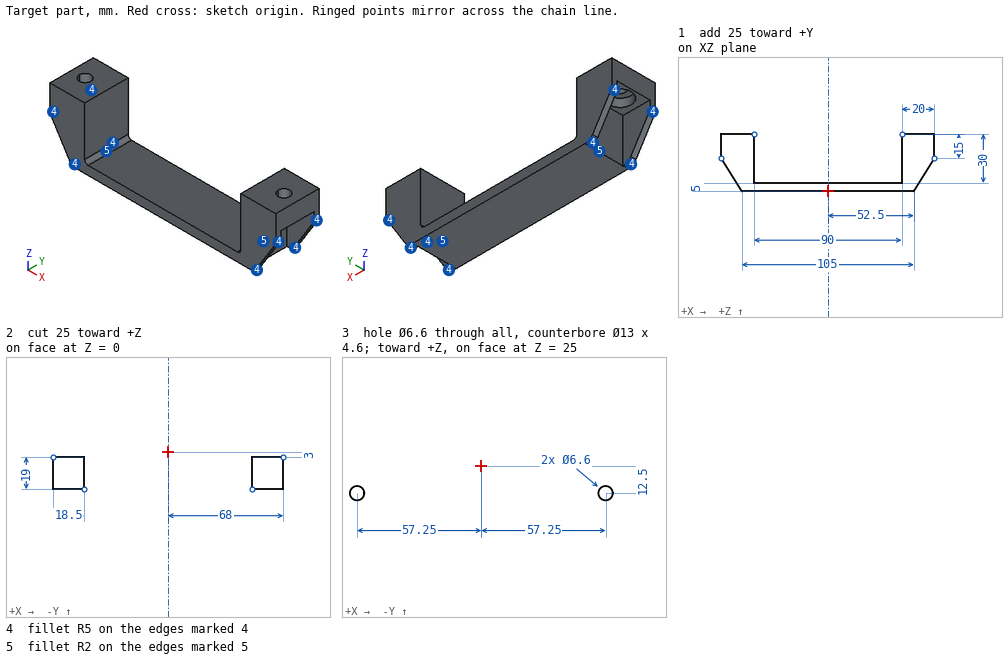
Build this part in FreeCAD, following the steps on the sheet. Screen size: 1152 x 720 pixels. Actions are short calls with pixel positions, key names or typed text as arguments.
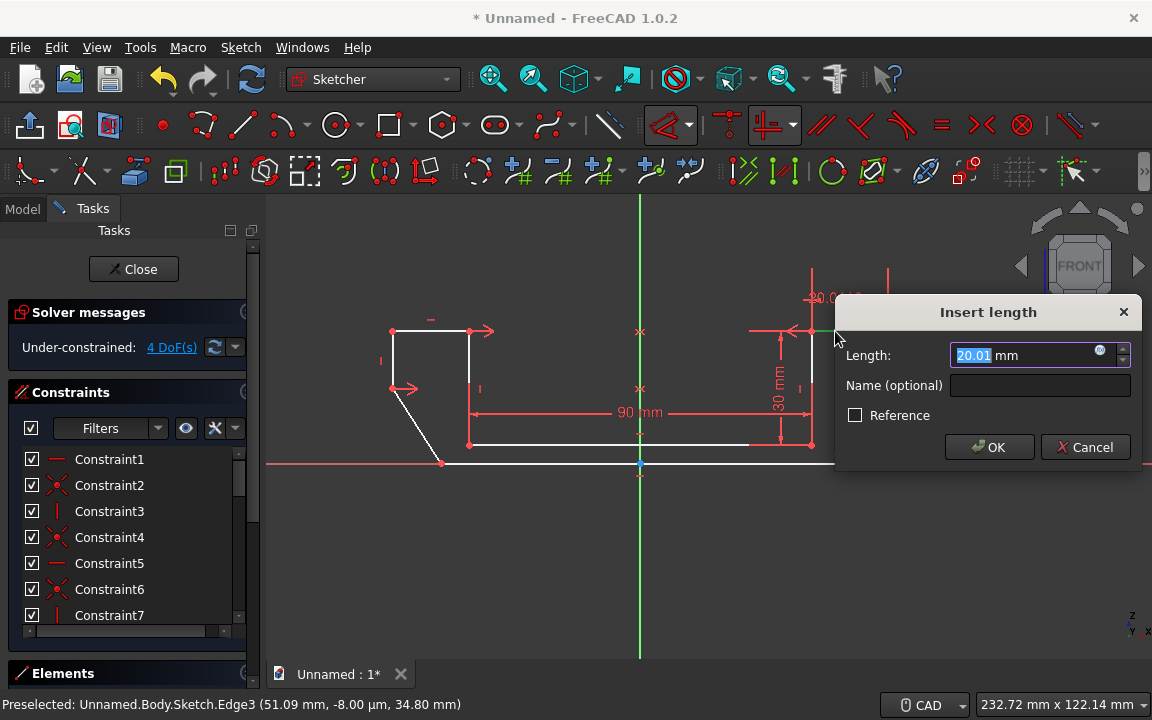
text(20)
key(Return)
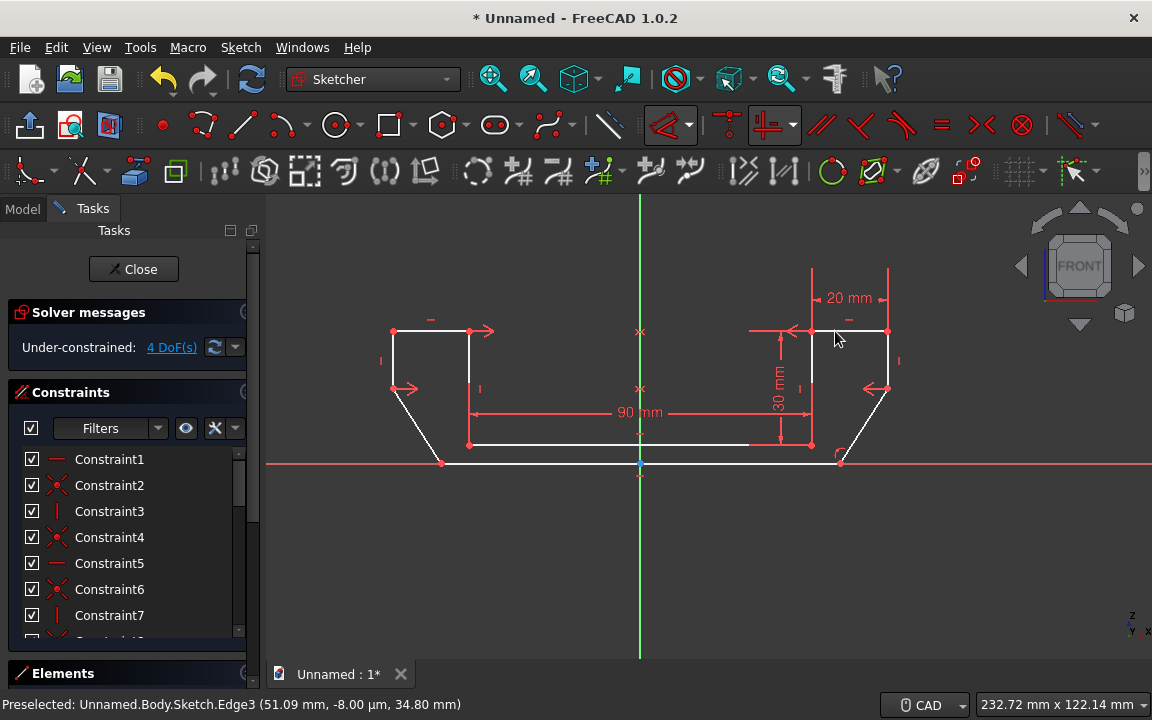
click(888, 349)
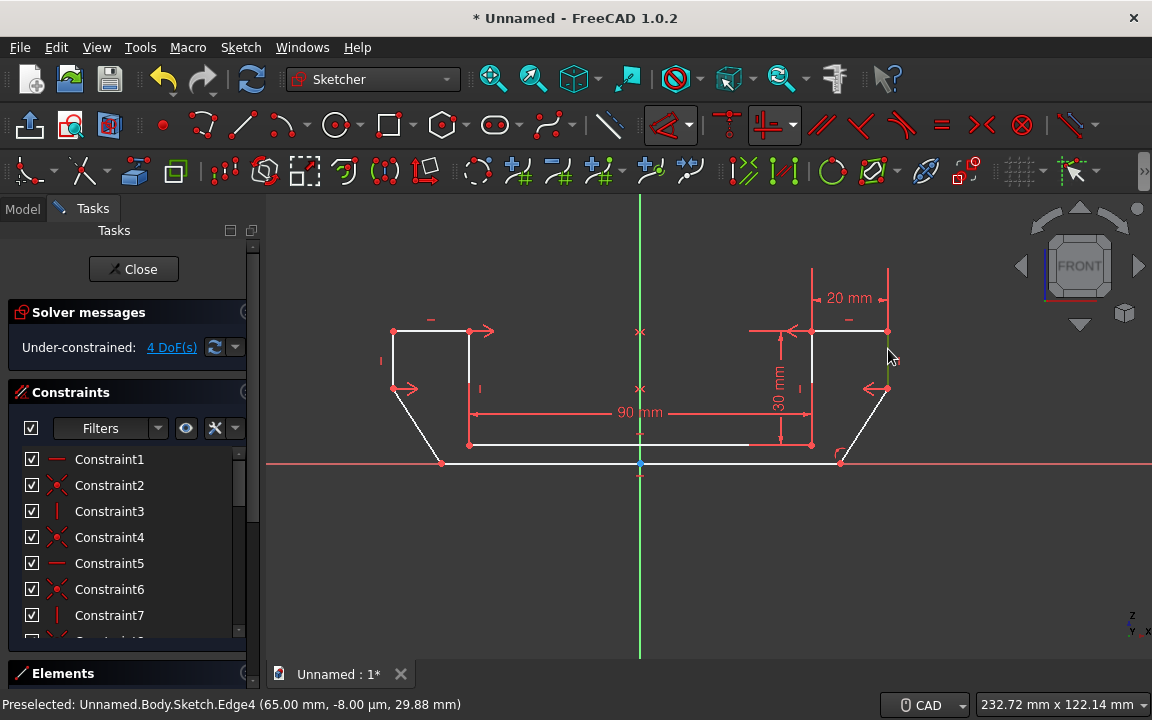
key(i)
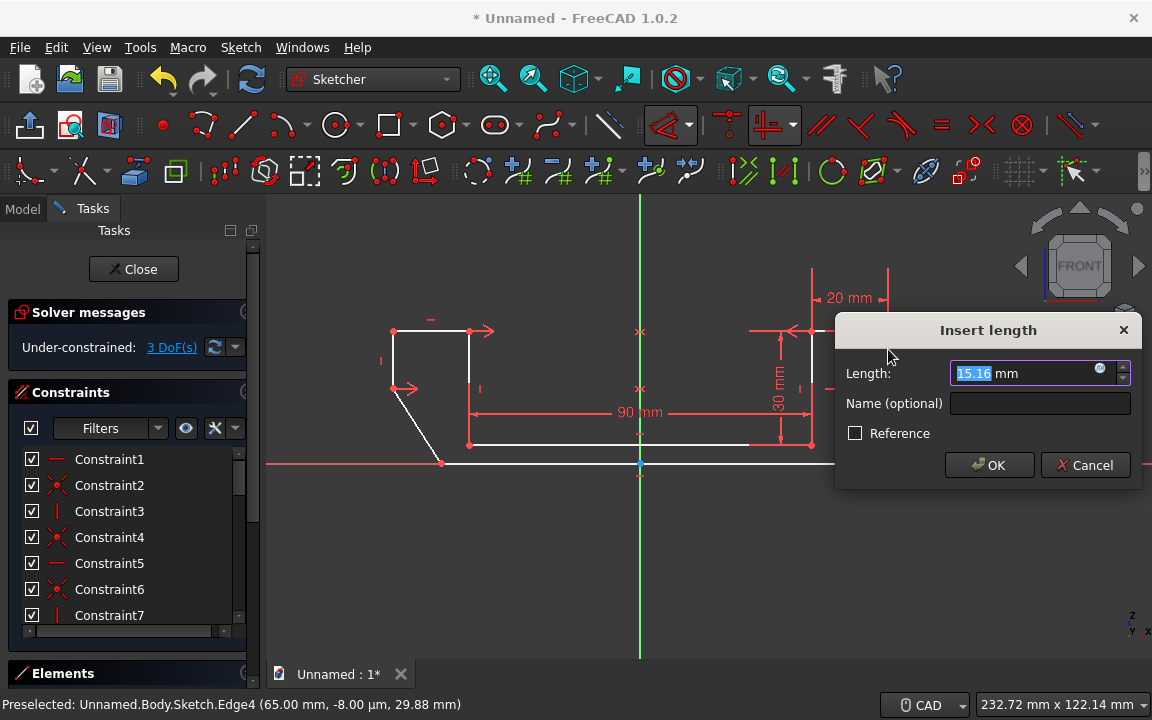
text(15)
key(Return)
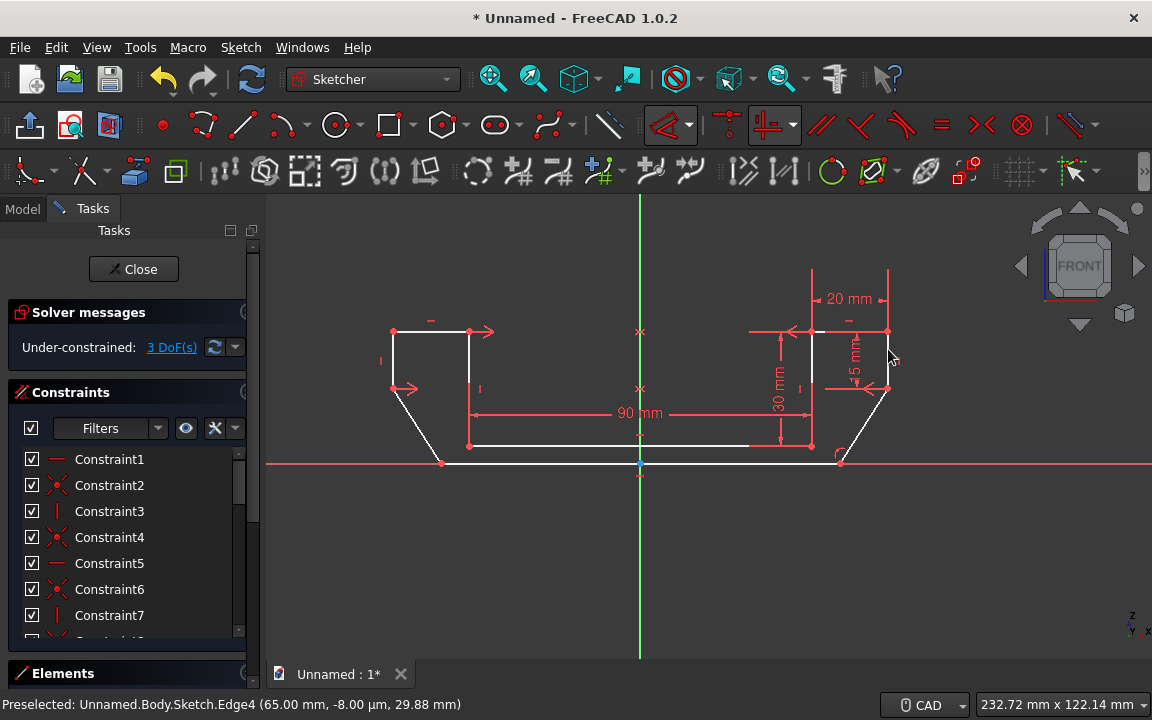
scroll(469, 446, up, 4)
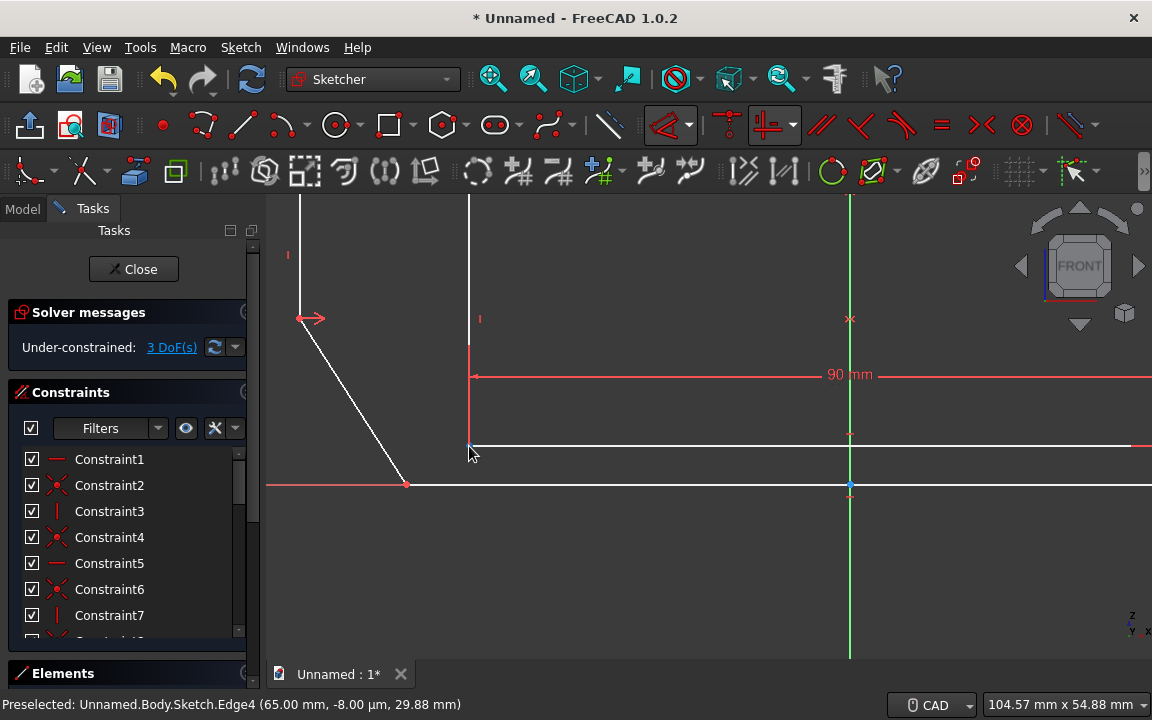
click(469, 446)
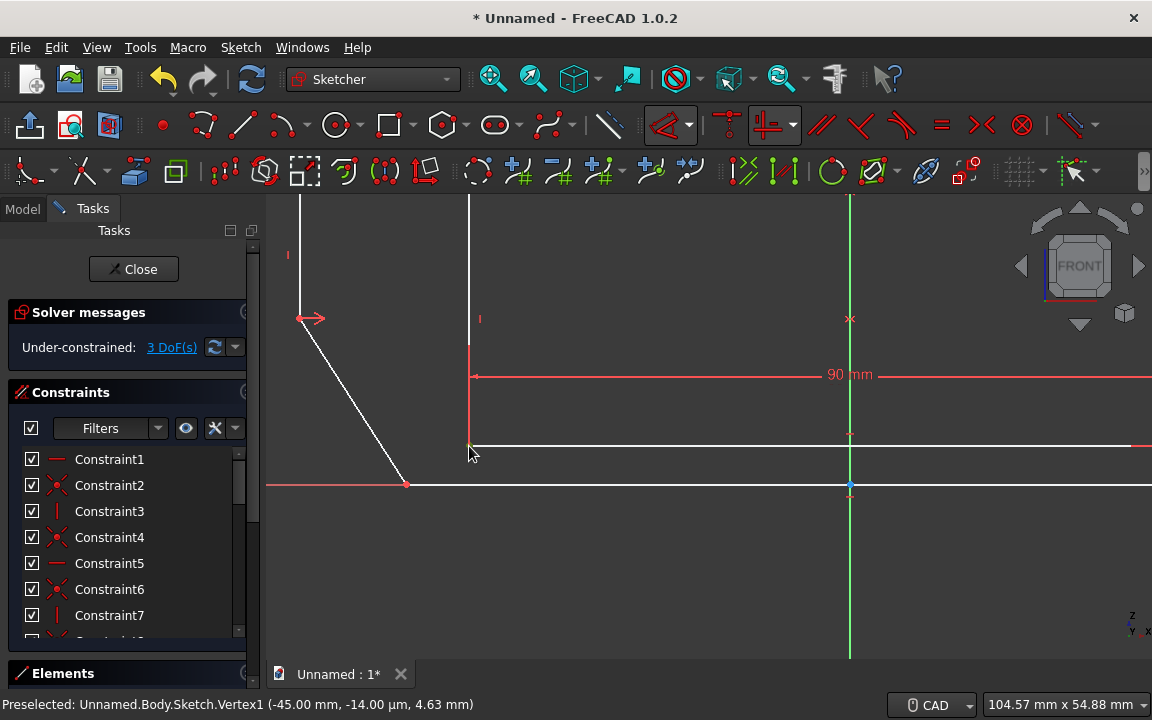
key(i)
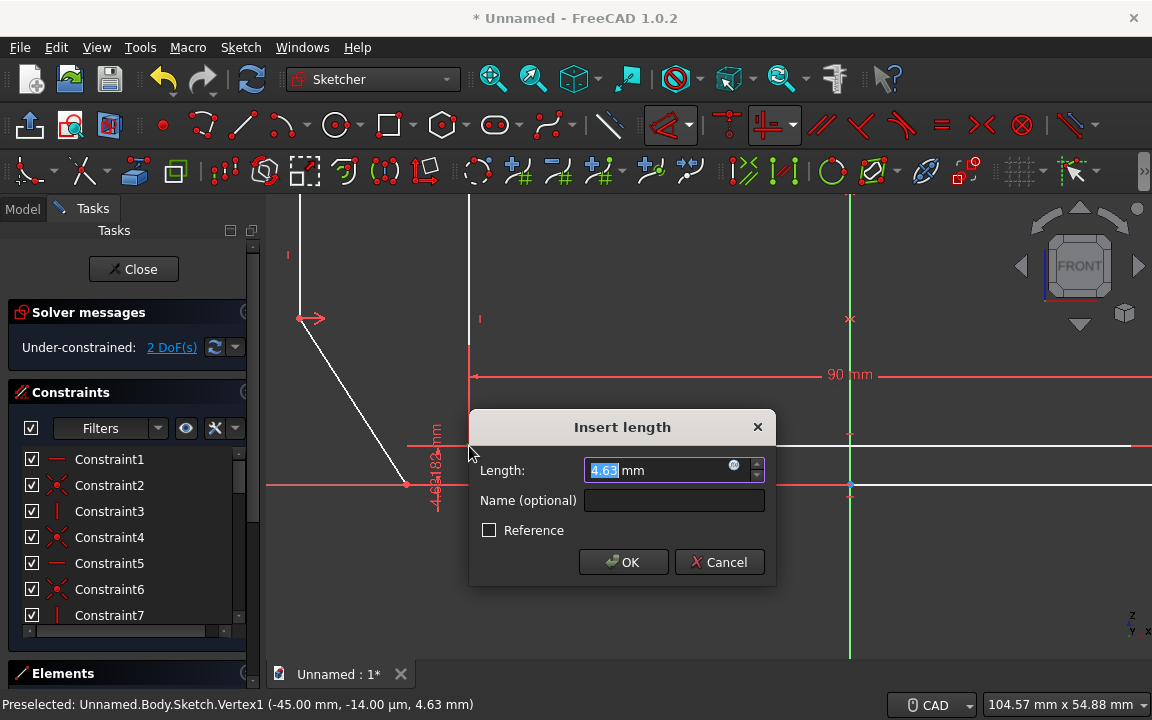
text(5)
key(Return)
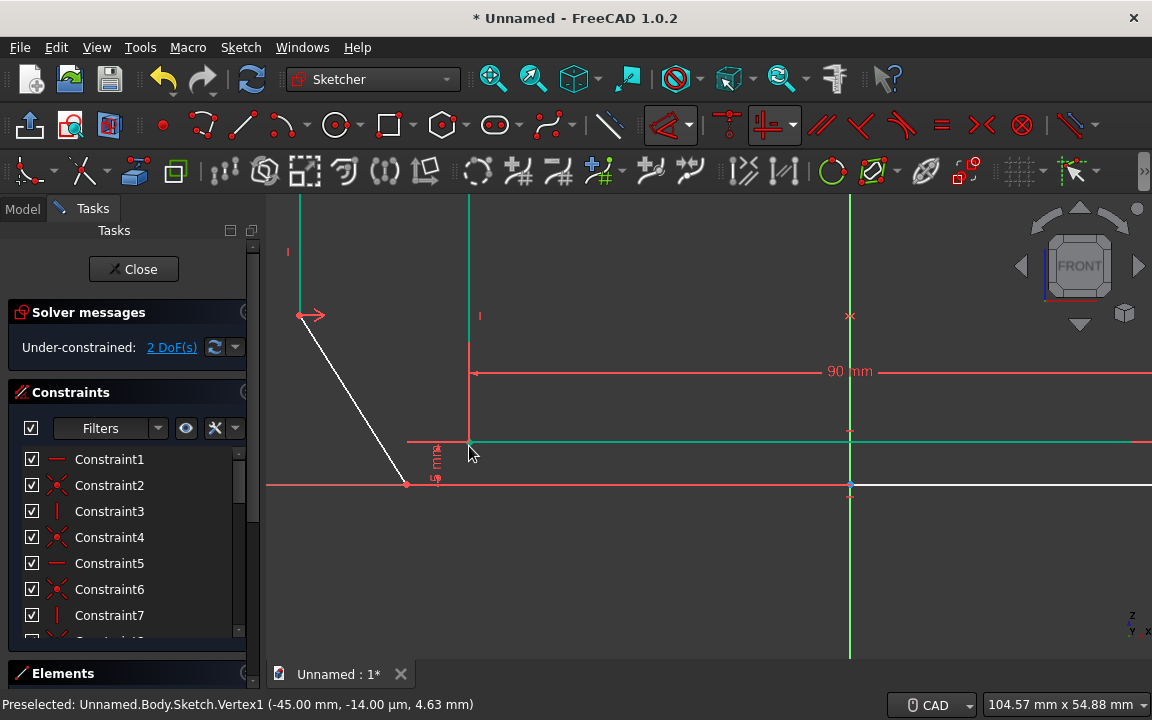
click(673, 485)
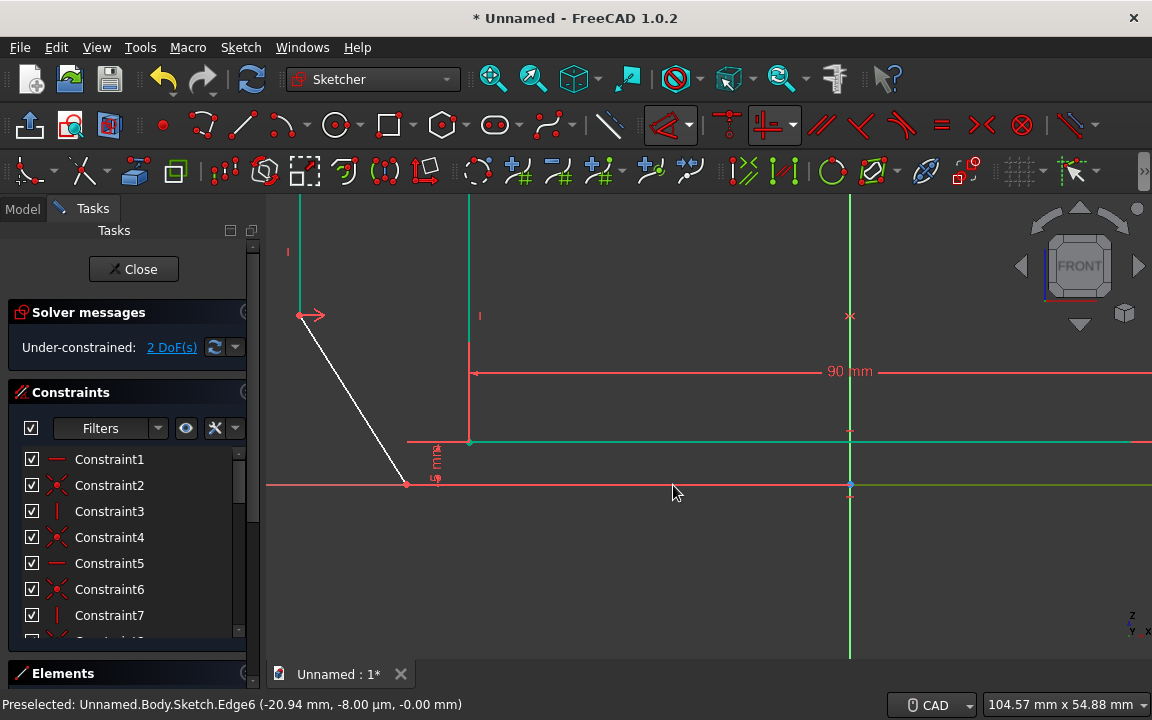
click(692, 126)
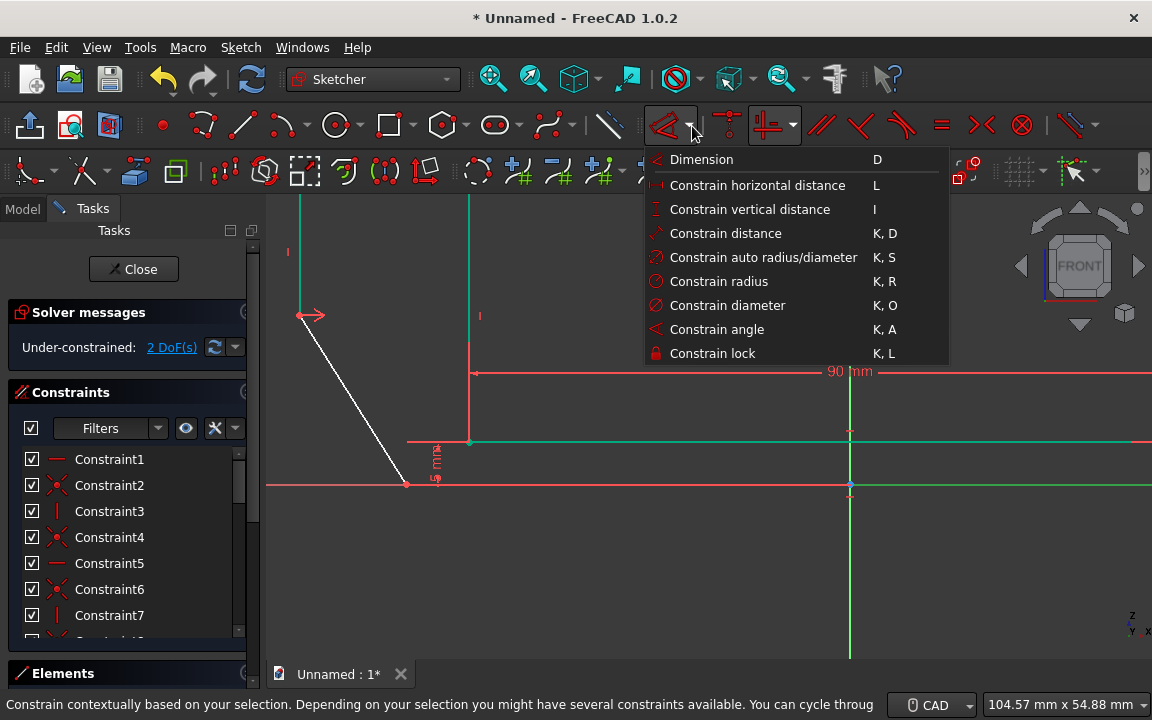
click(797, 185)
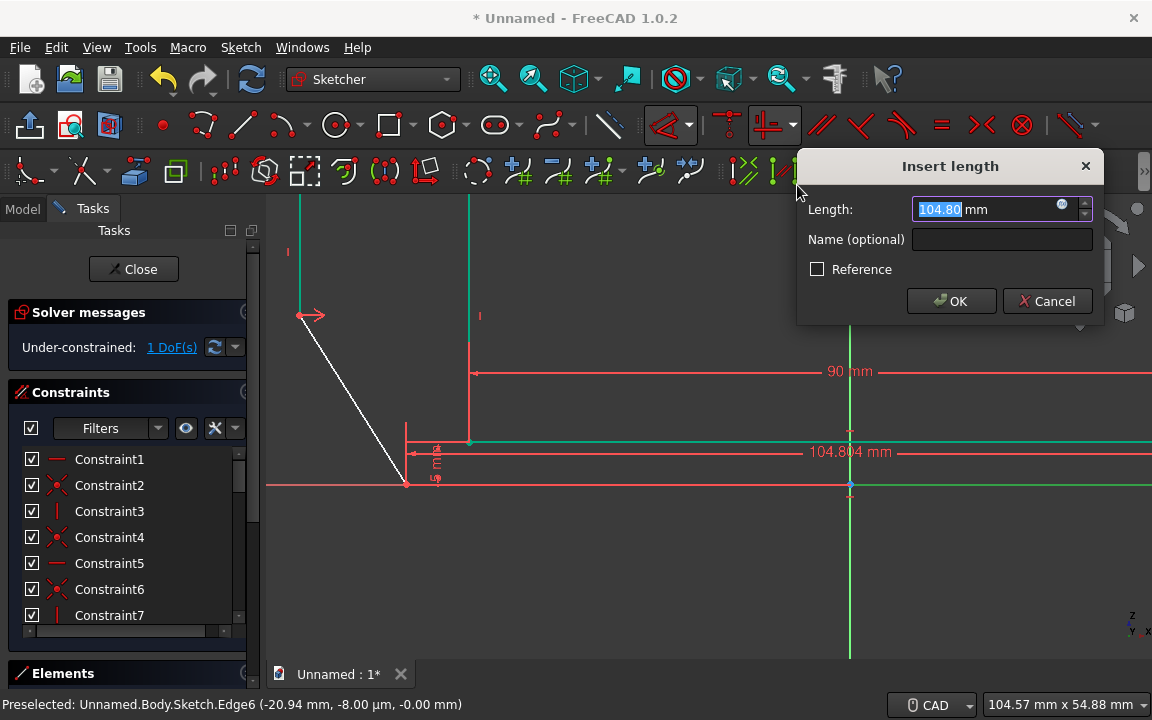
text(105)
key(Return)